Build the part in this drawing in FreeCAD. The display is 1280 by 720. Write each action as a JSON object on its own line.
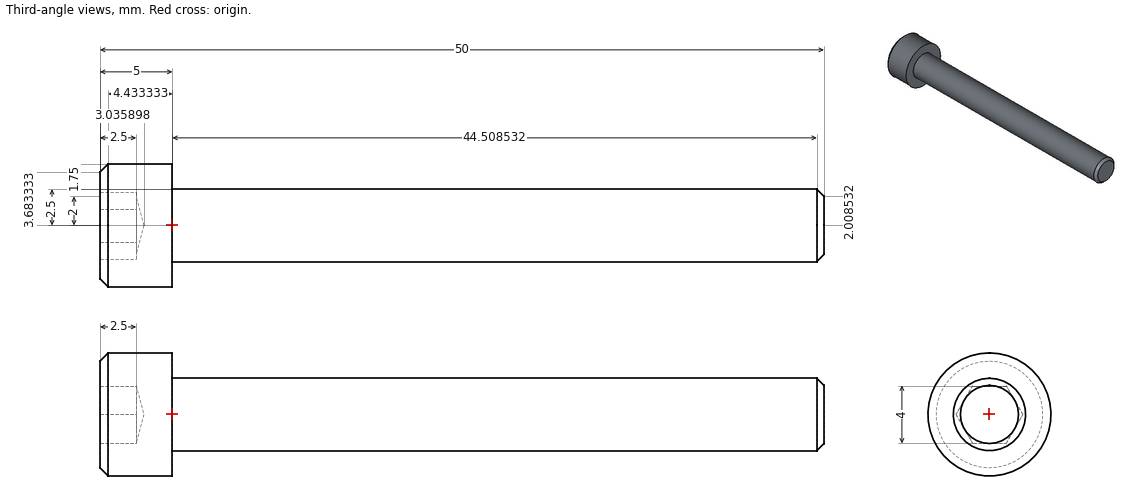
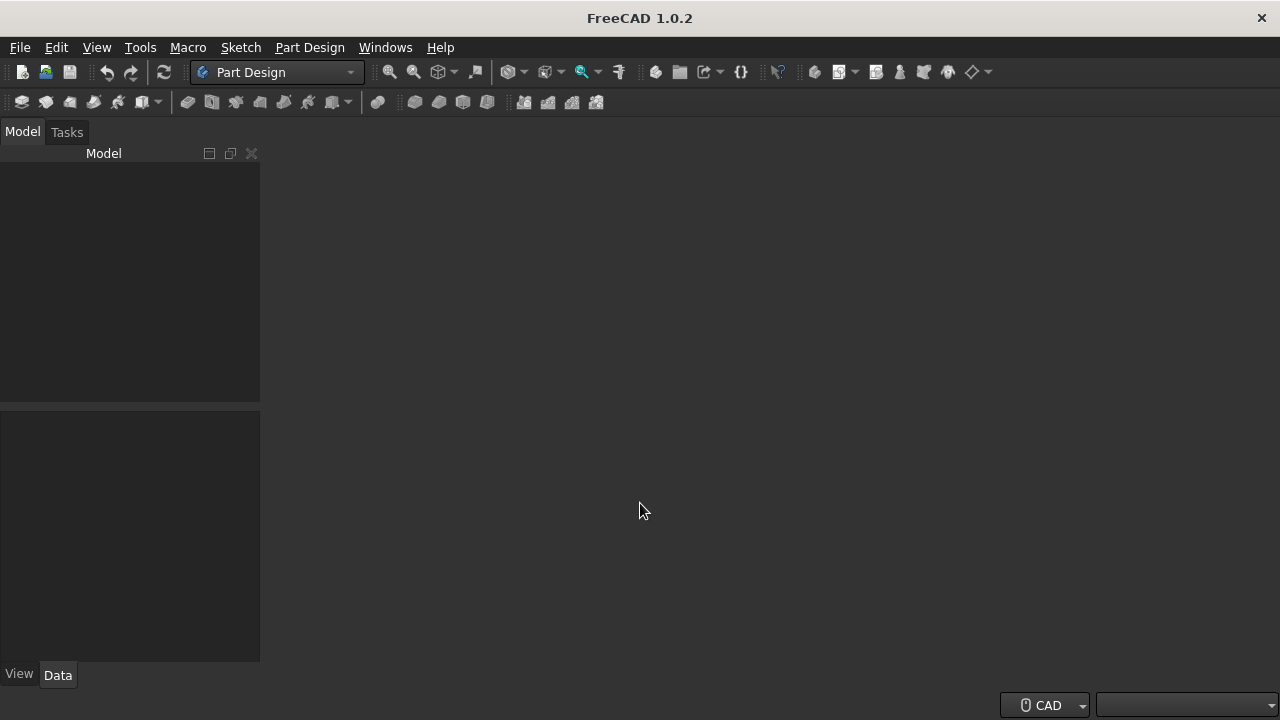
{"action": "key", "text": "ctrl+n"}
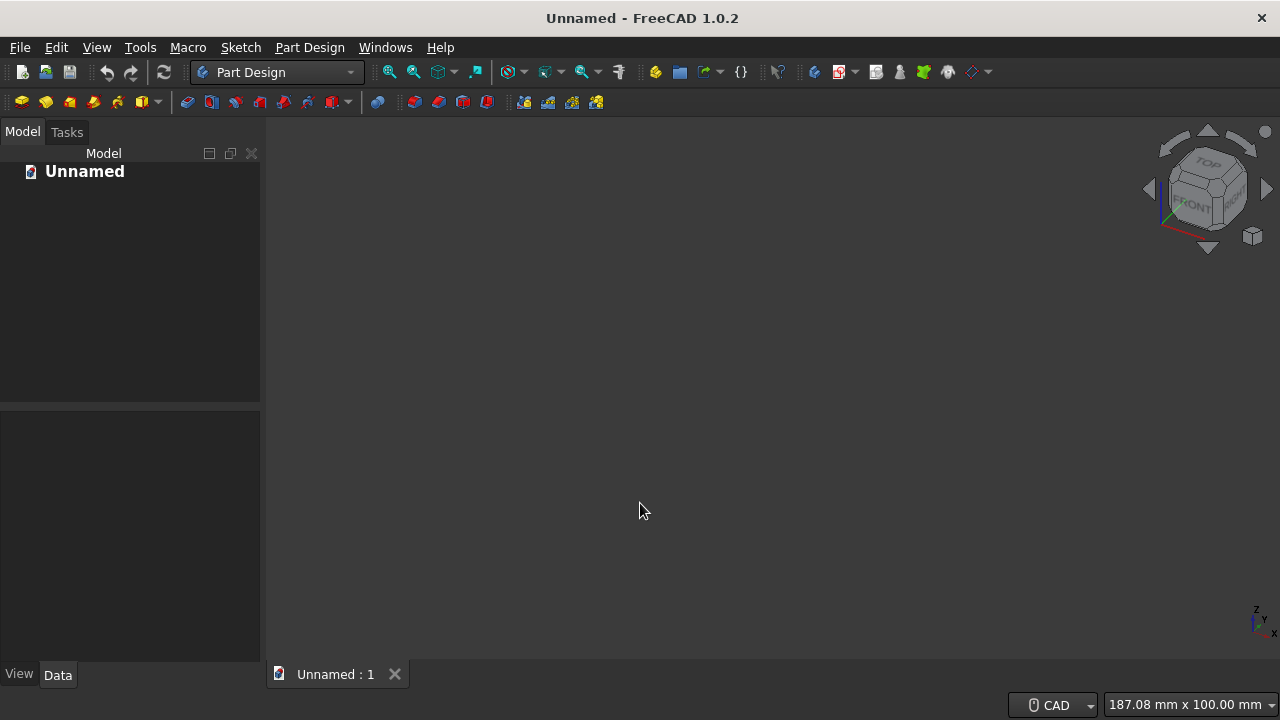
{"action": "left_click", "coordinate": [840, 72]}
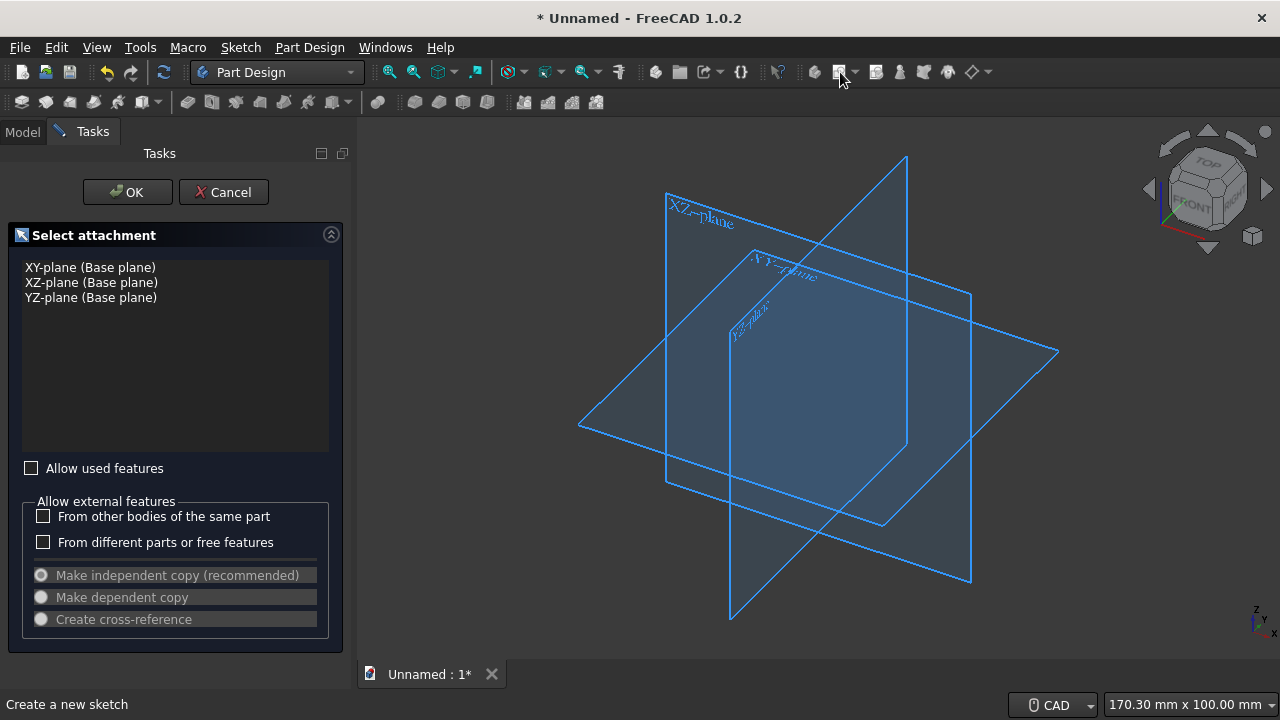
{"action": "left_click", "coordinate": [82, 268]}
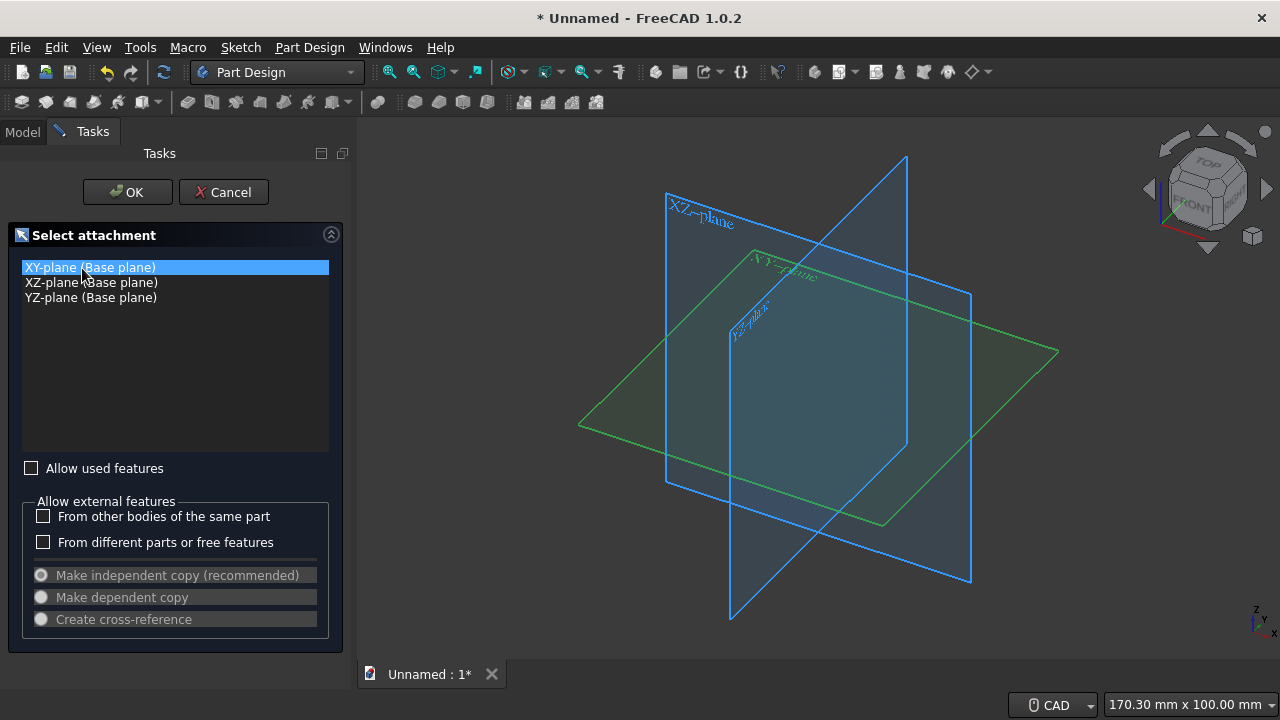
{"action": "left_click", "coordinate": [128, 192]}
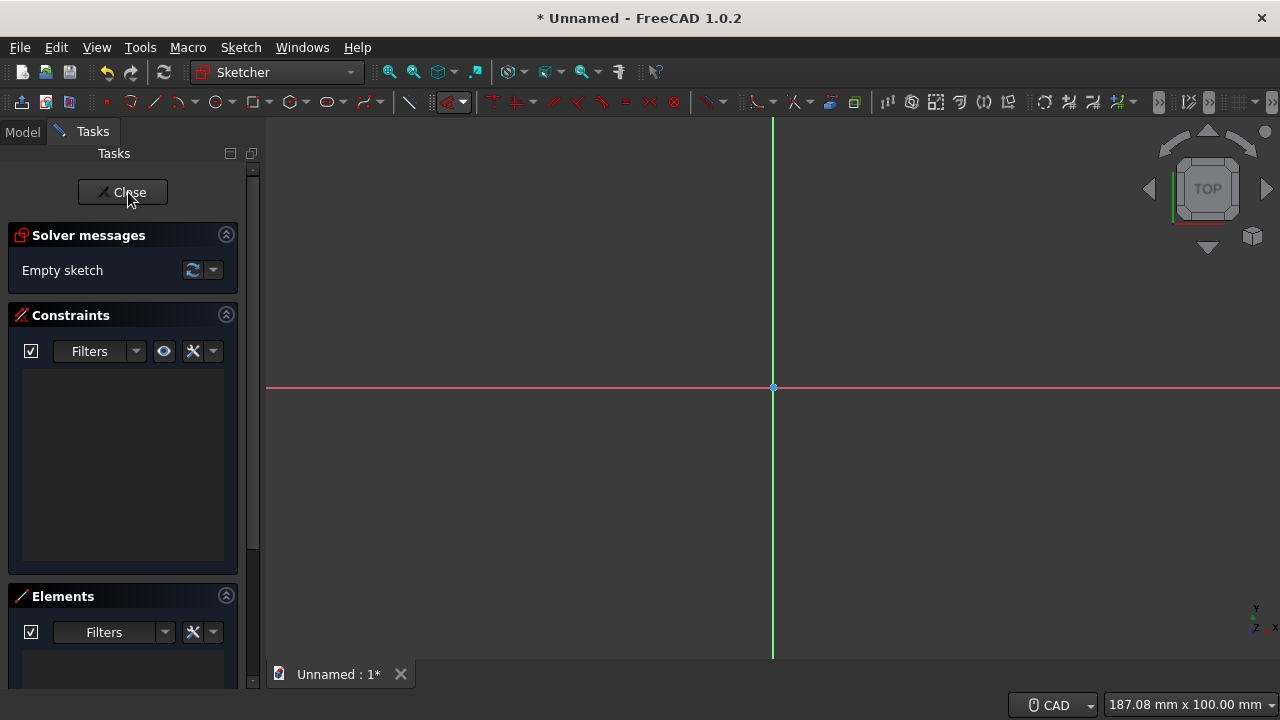
{"action": "scroll", "coordinate": [1026, 367], "scroll_direction": "up", "scroll_amount": 4}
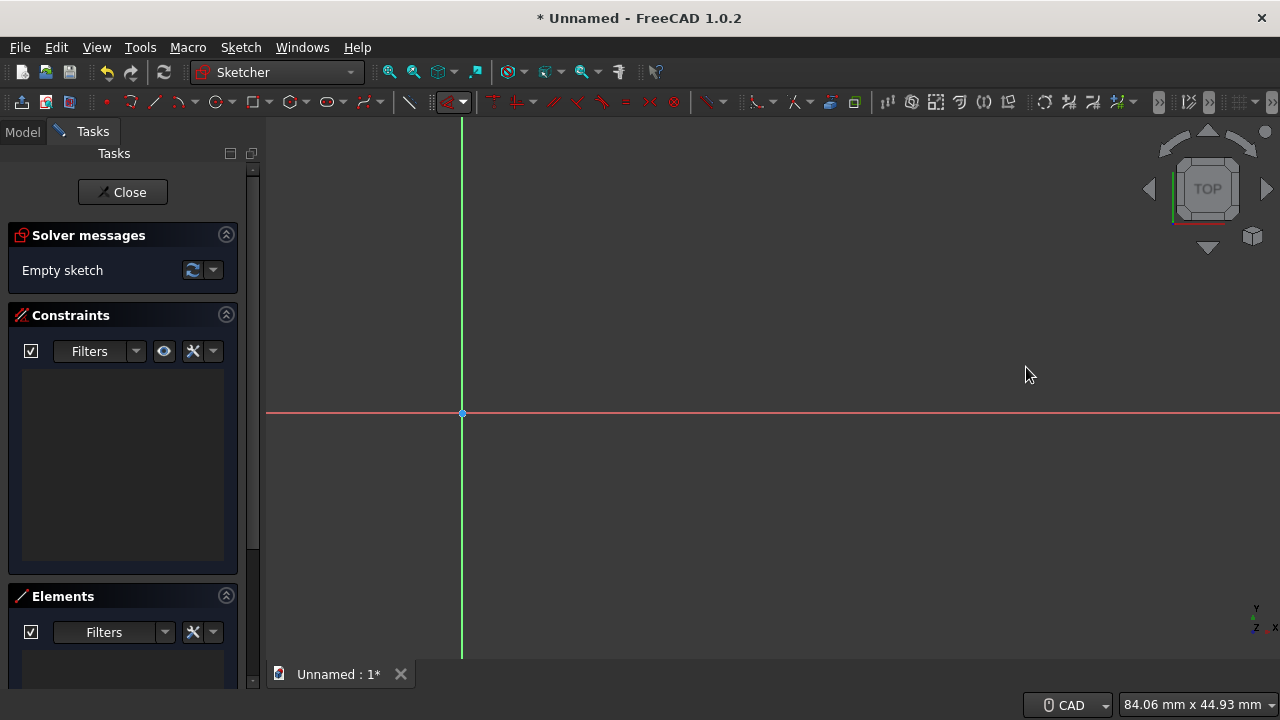
{"action": "key", "text": "g m"}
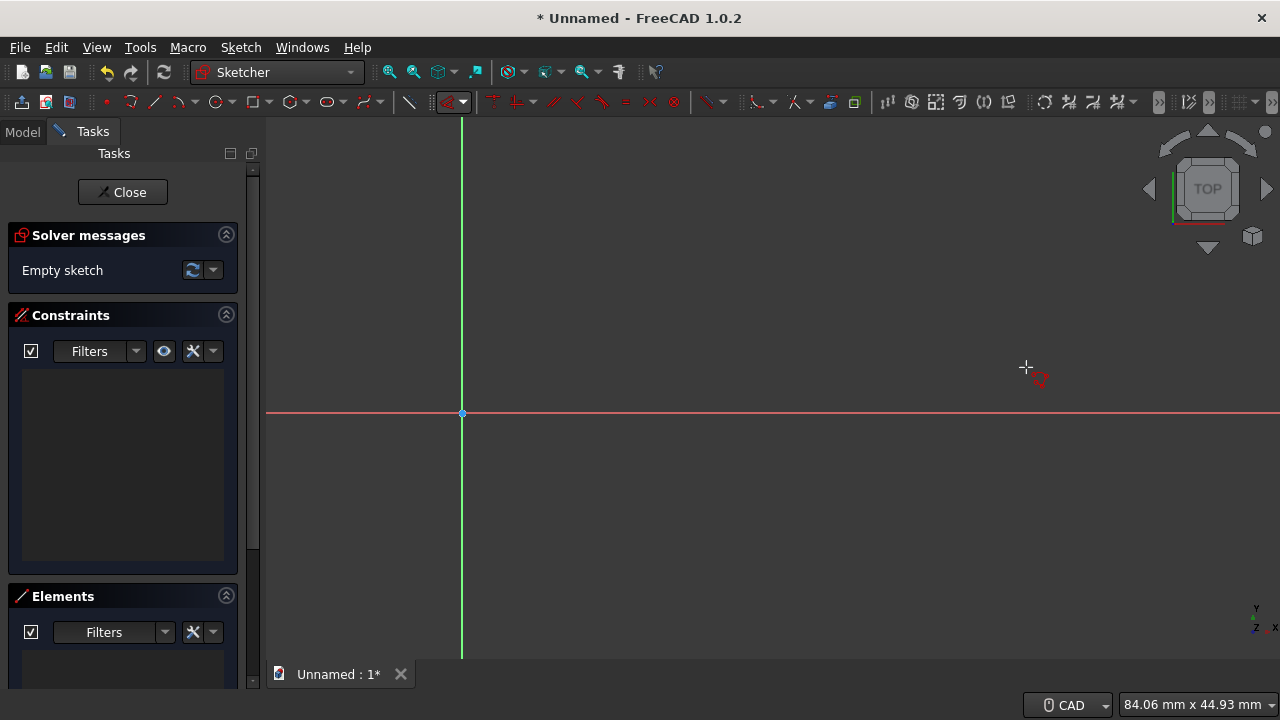
{"action": "left_click", "coordinate": [462, 383]}
{"action": "left_click", "coordinate": [471, 362]}
{"action": "left_click", "coordinate": [409, 362]}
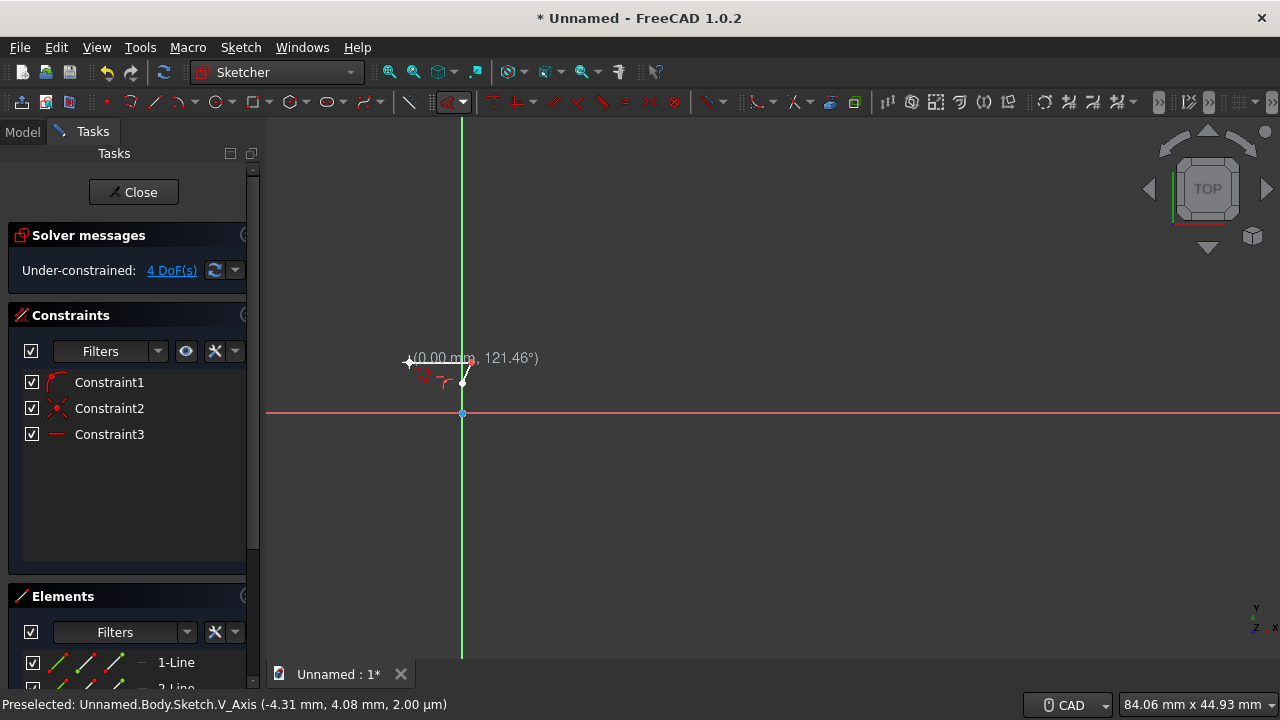
{"action": "scroll", "coordinate": [402, 369], "scroll_direction": "up", "scroll_amount": 3}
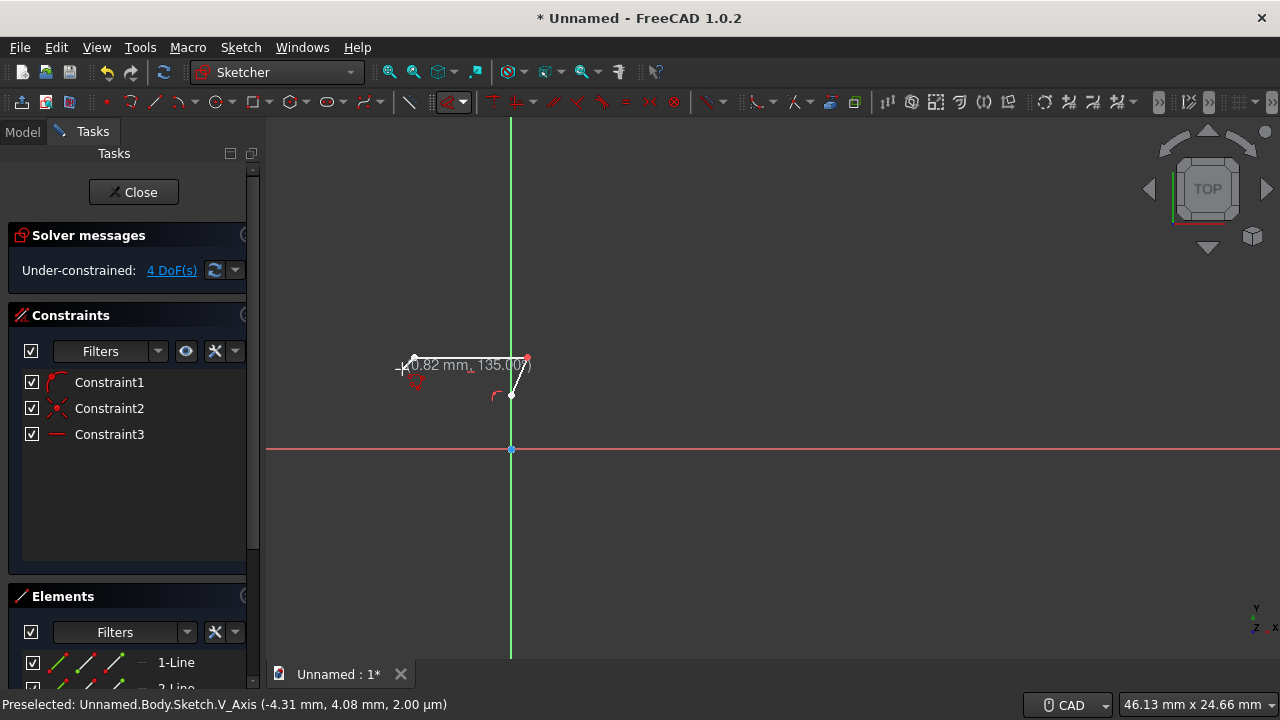
{"action": "left_click", "coordinate": [401, 368]}
{"action": "left_click", "coordinate": [401, 449]}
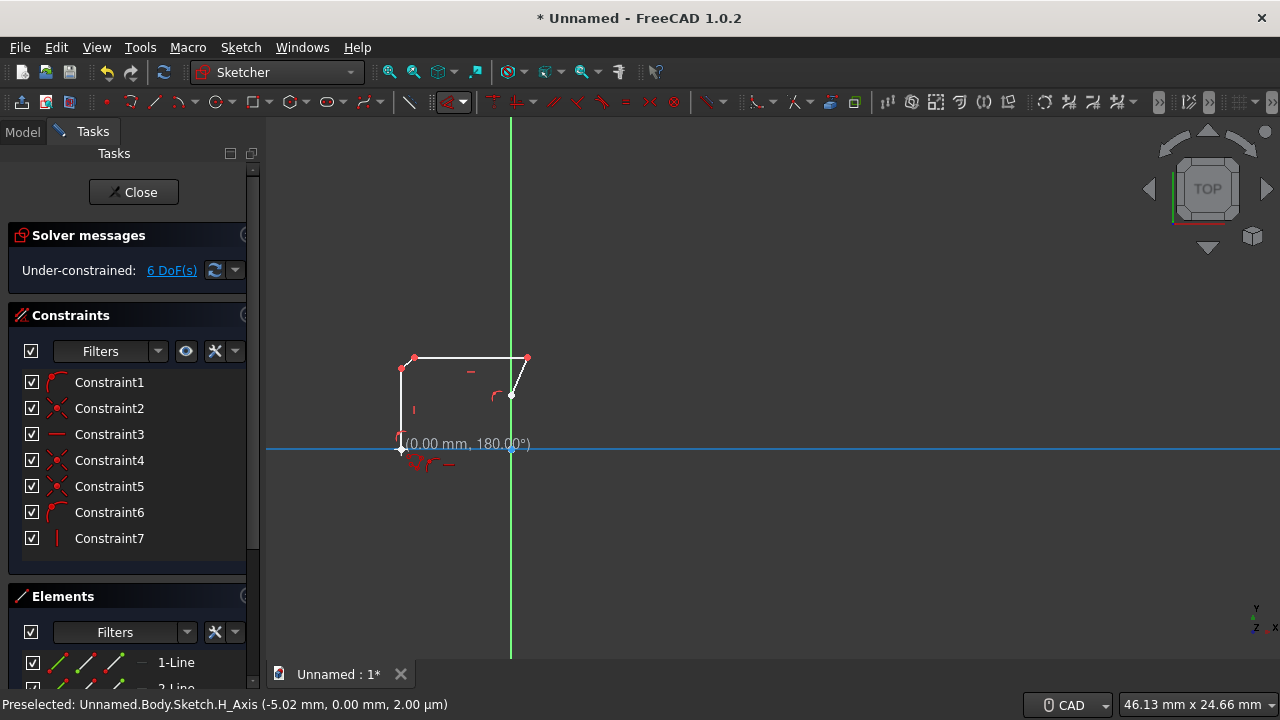
{"action": "scroll", "coordinate": [405, 370], "scroll_direction": "down", "scroll_amount": 3}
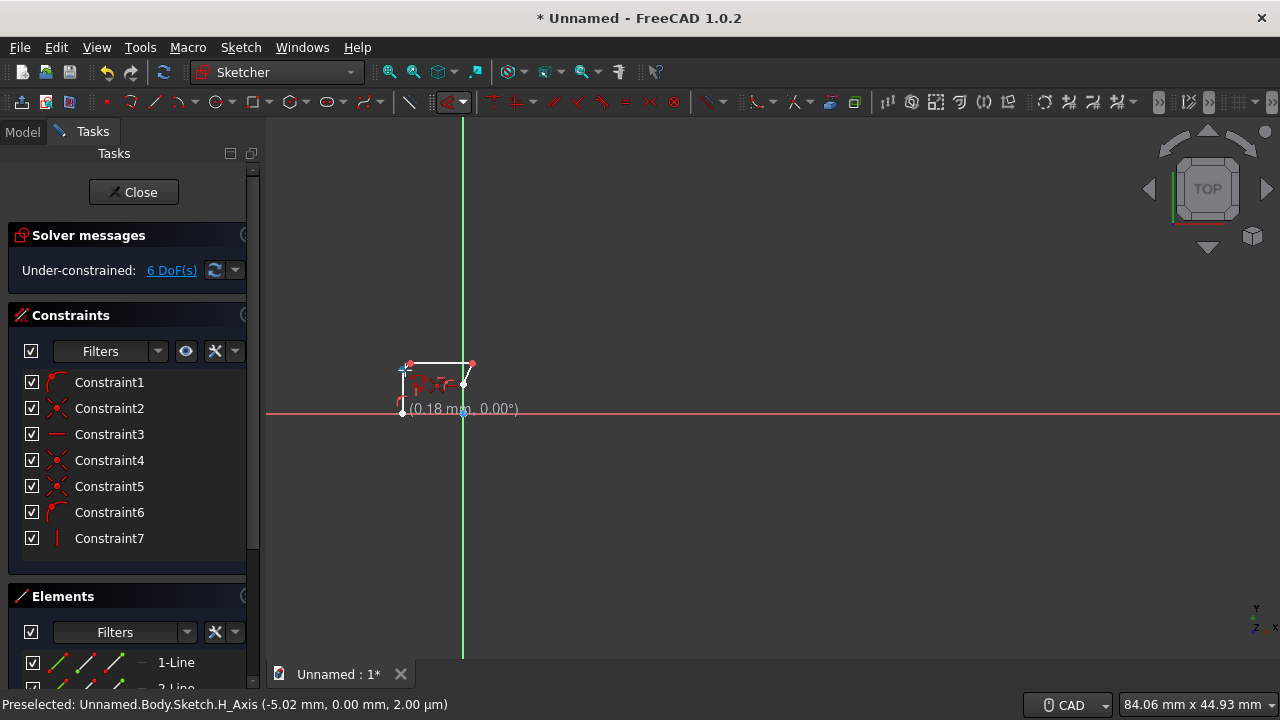
{"action": "left_click", "coordinate": [1006, 405]}
{"action": "left_click", "coordinate": [1006, 389]}